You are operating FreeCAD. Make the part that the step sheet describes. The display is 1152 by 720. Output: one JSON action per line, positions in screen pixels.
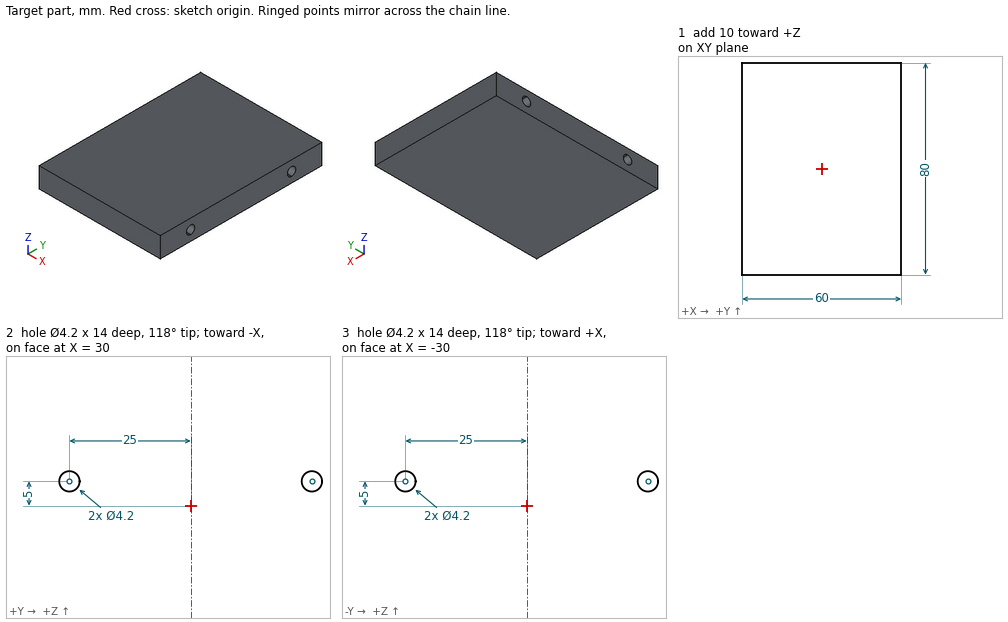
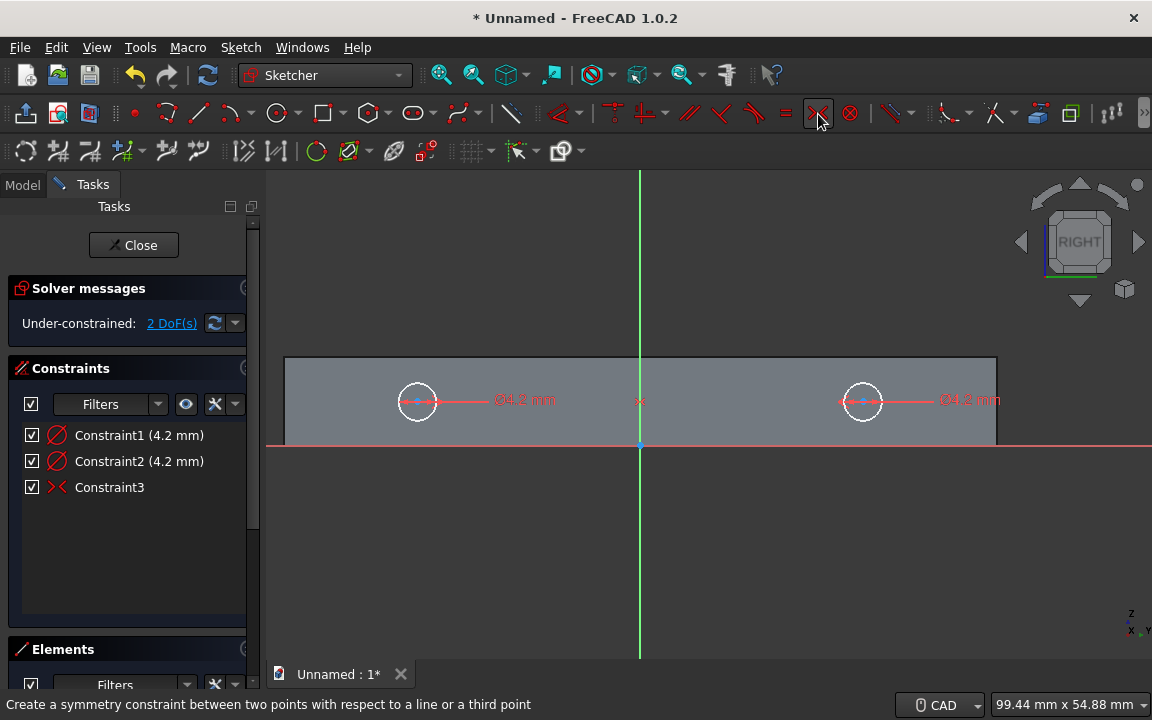
{"action": "left_click", "coordinate": [418, 402]}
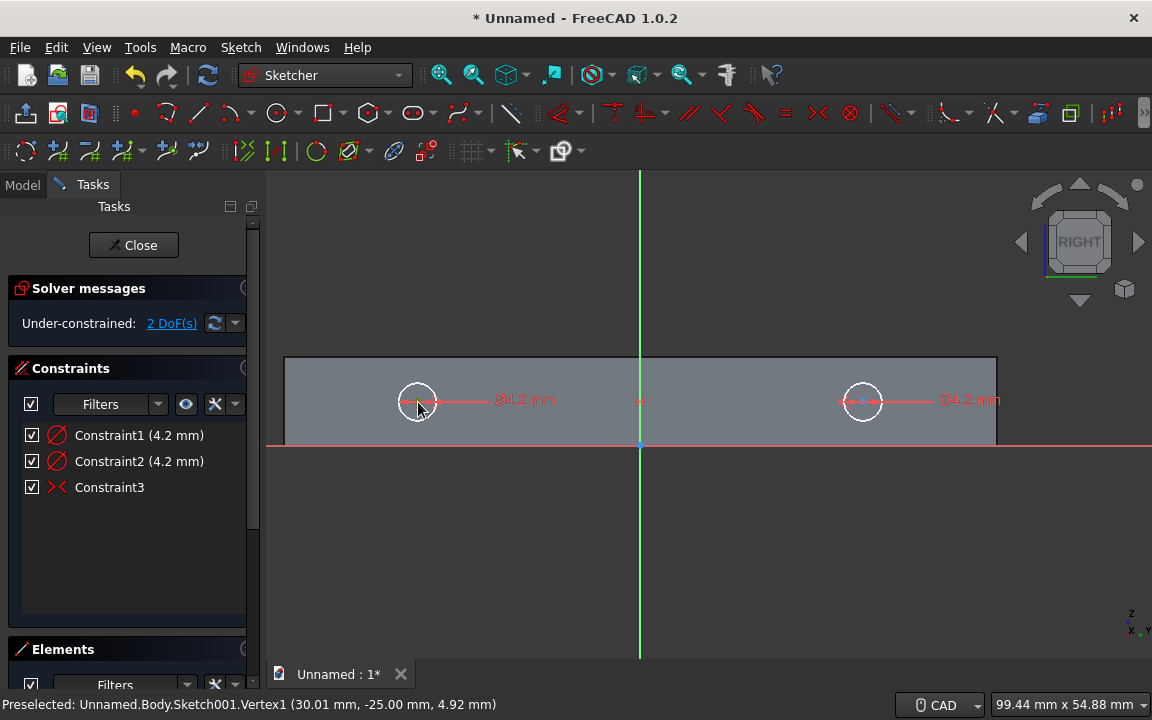
{"action": "key", "text": "i"}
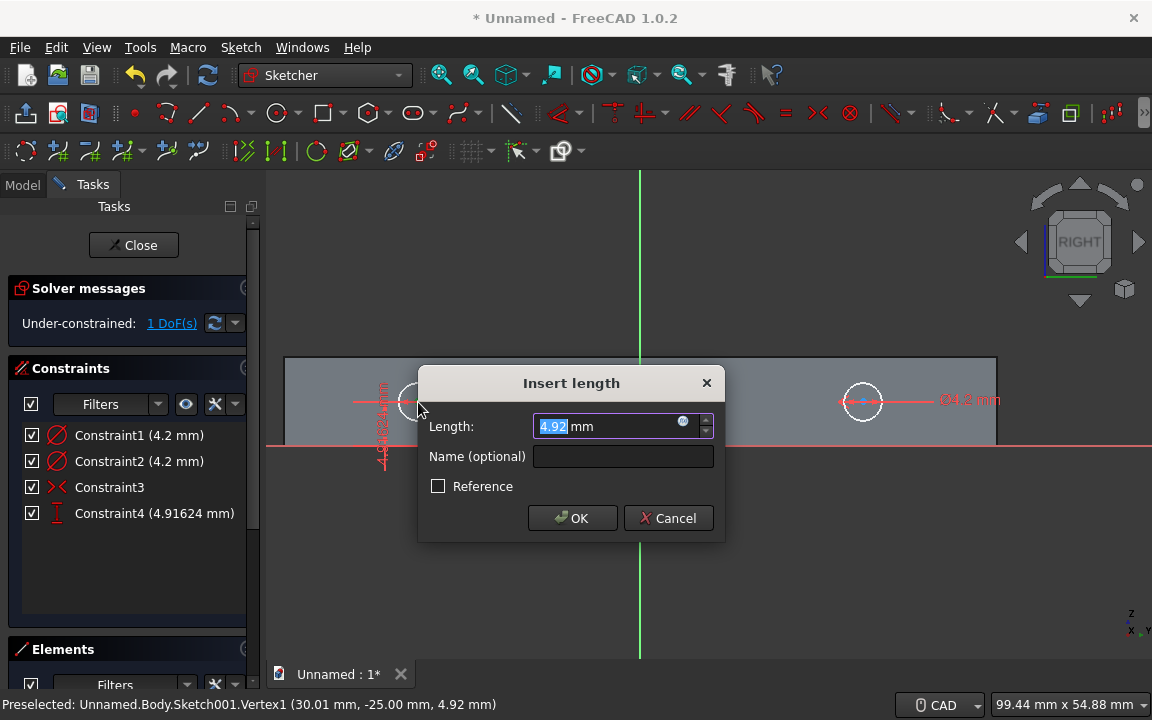
{"action": "type", "text": "5"}
{"action": "key", "text": "Return"}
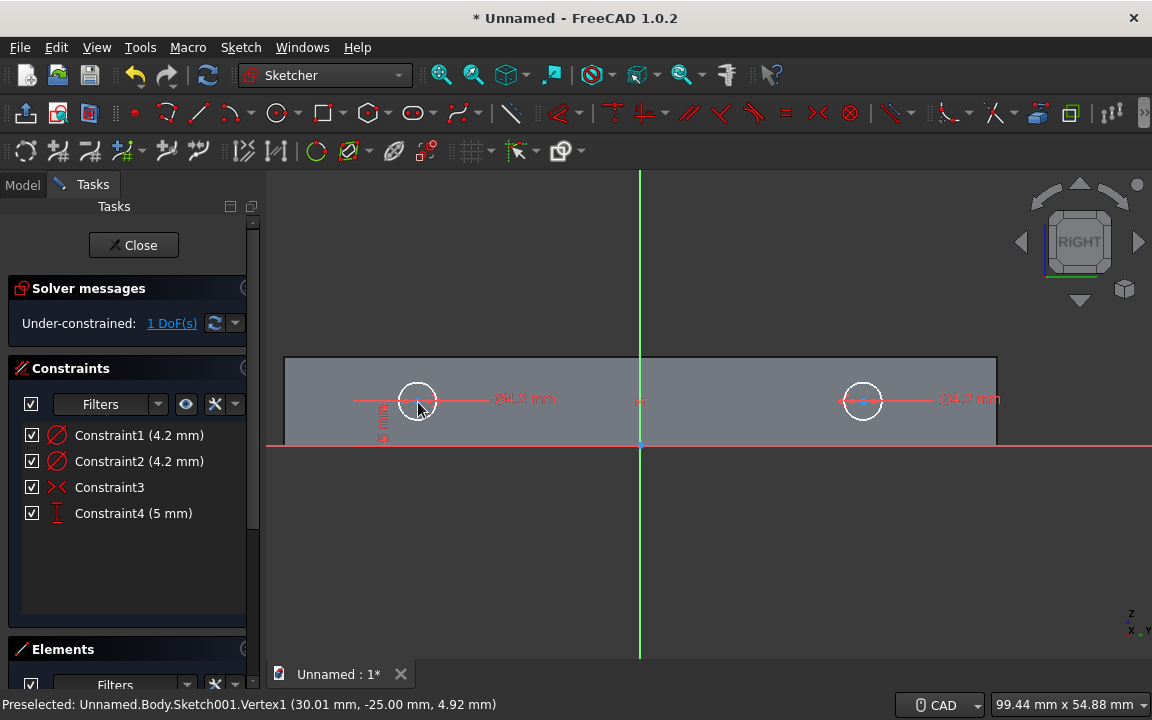
{"action": "left_click", "coordinate": [418, 401]}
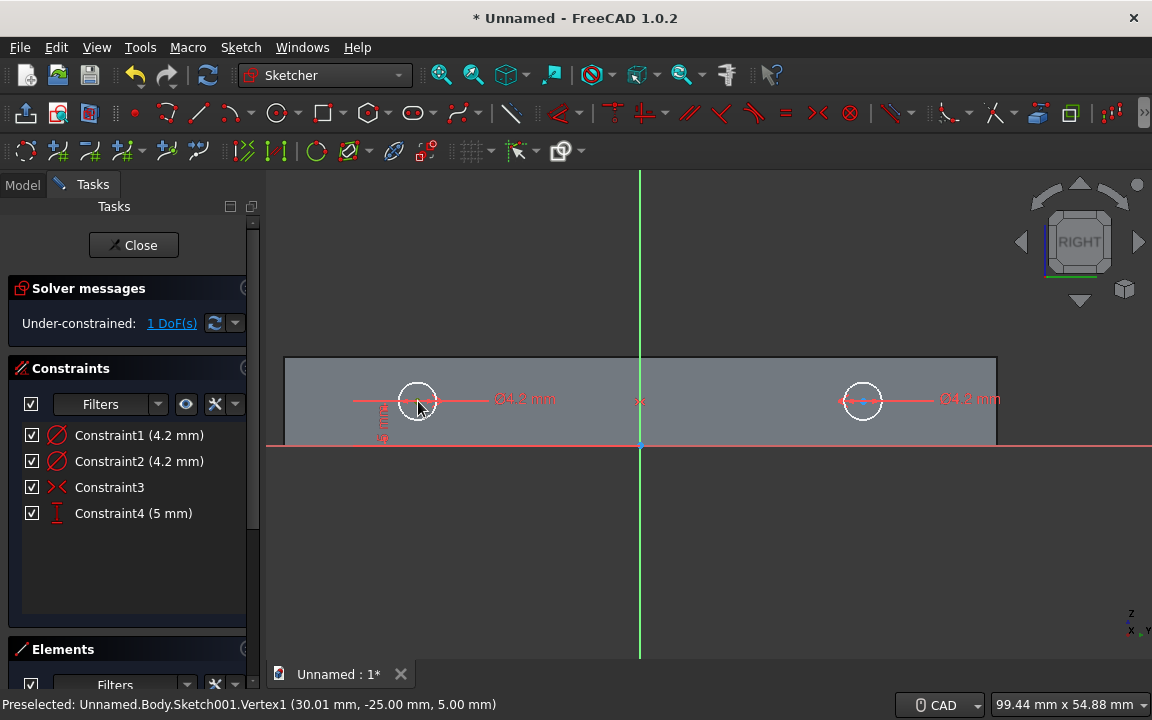
{"action": "left_click", "coordinate": [582, 114]}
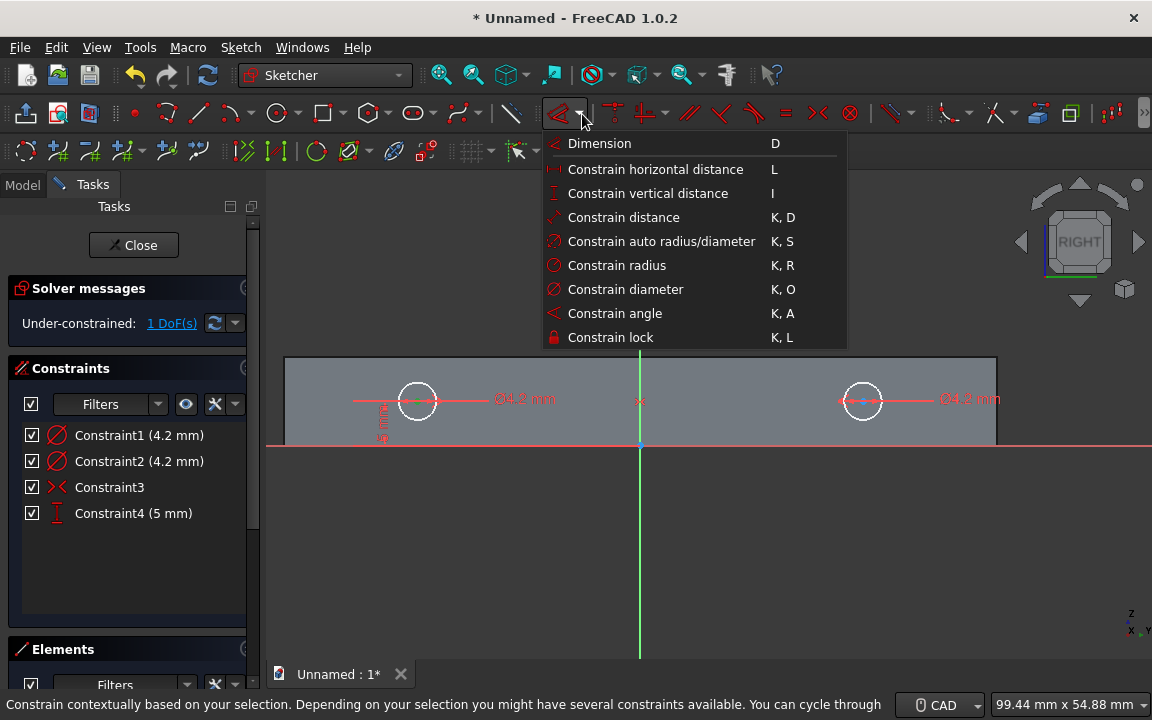
{"action": "left_click", "coordinate": [695, 169]}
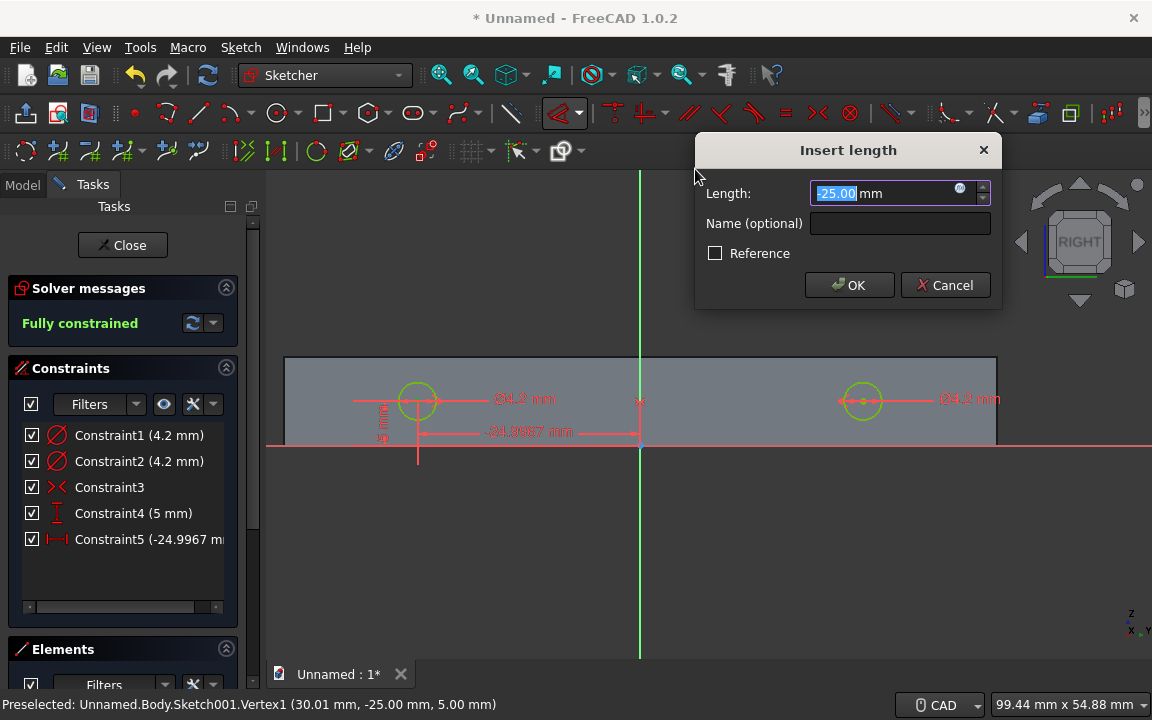
{"action": "type", "text": "-25"}
{"action": "key", "text": "Return"}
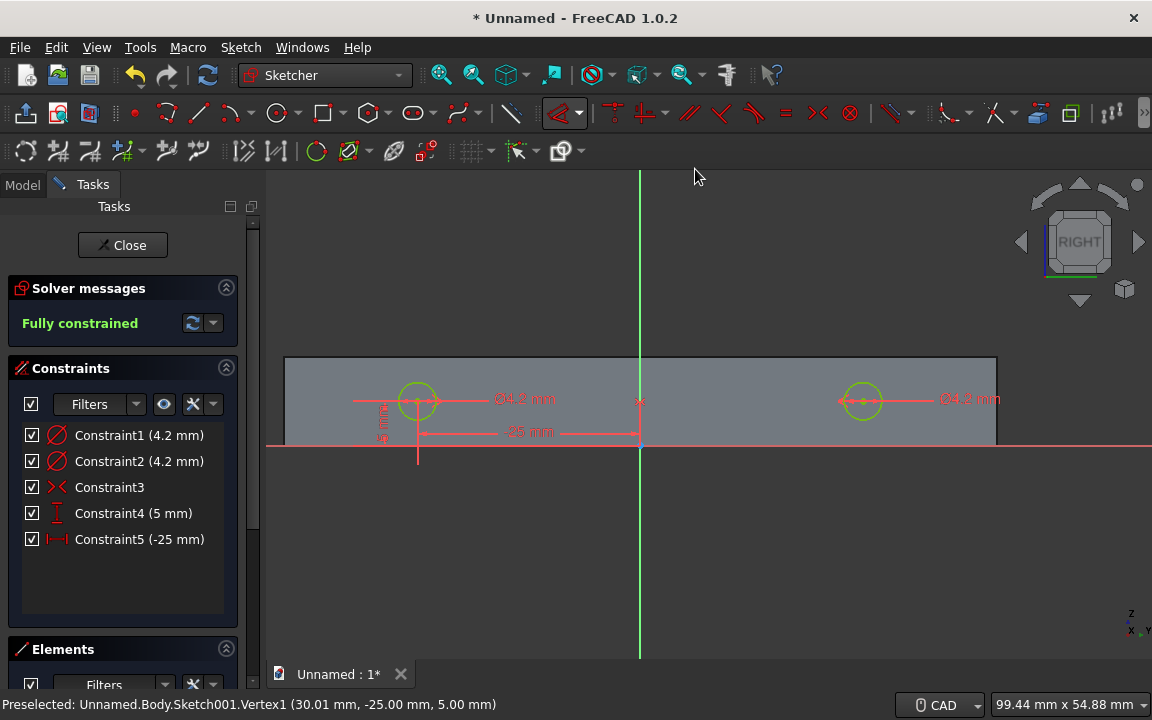
{"action": "left_click", "coordinate": [123, 245]}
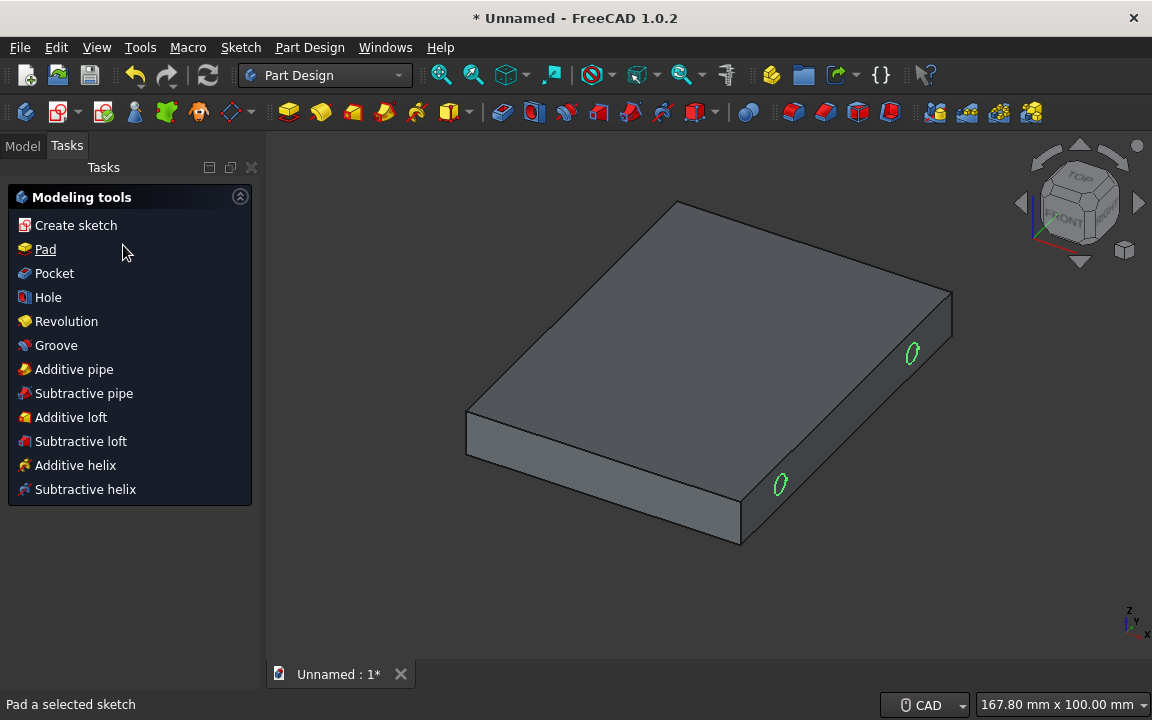
{"action": "left_click", "coordinate": [536, 112]}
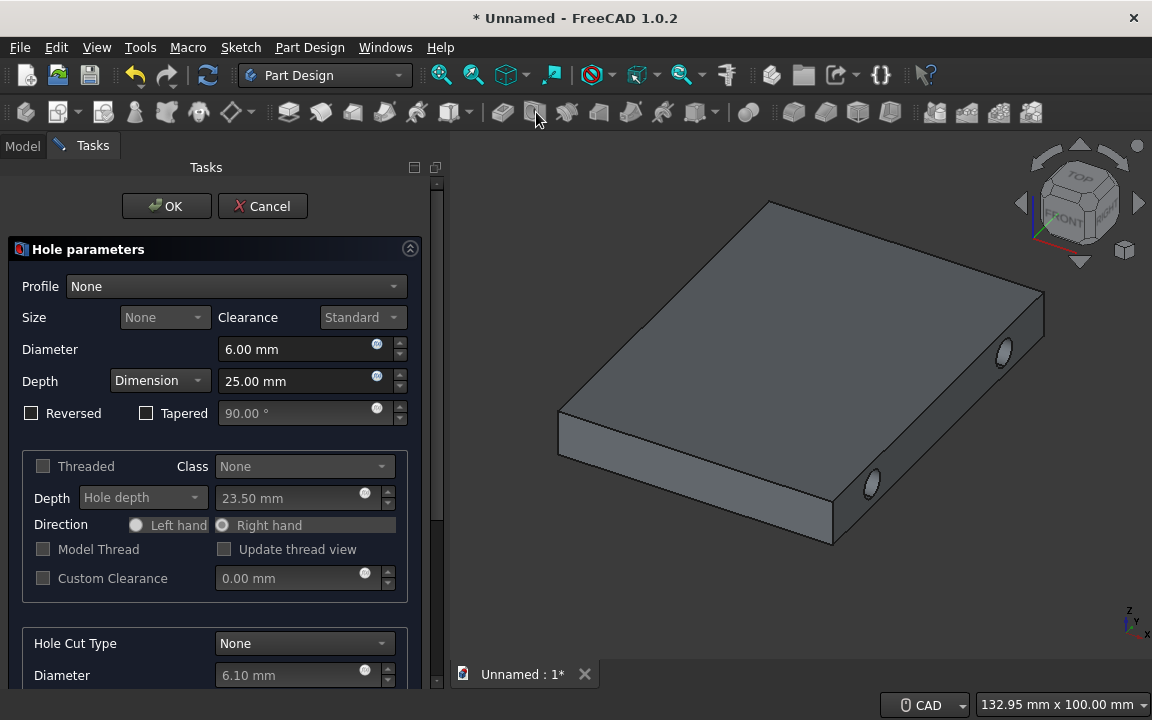
{"action": "triple_click", "coordinate": [305, 349]}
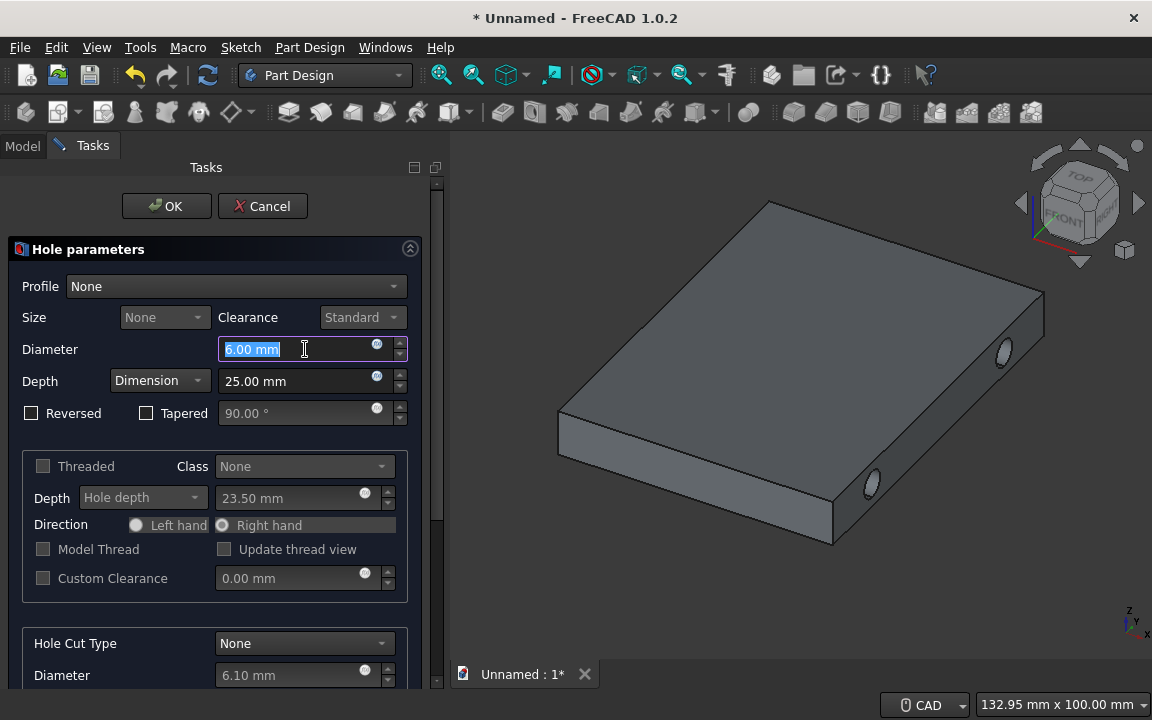
{"action": "type", "text": "4.2"}
{"action": "key", "text": "Tab"}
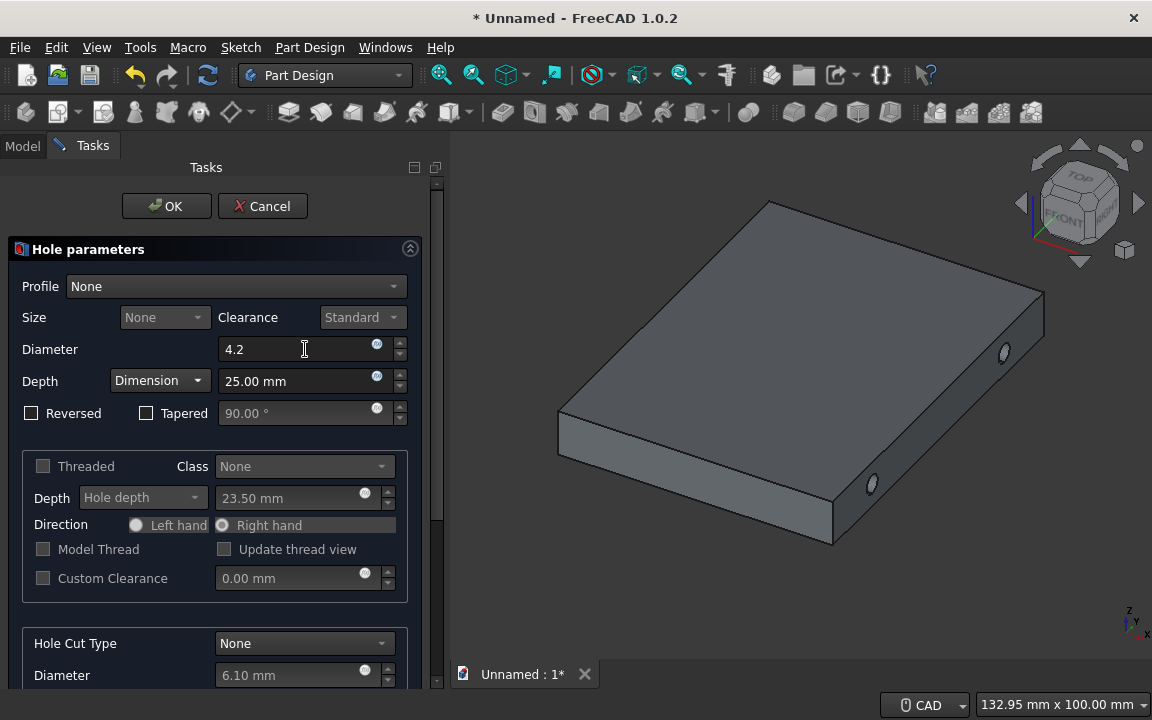
{"action": "triple_click", "coordinate": [305, 381]}